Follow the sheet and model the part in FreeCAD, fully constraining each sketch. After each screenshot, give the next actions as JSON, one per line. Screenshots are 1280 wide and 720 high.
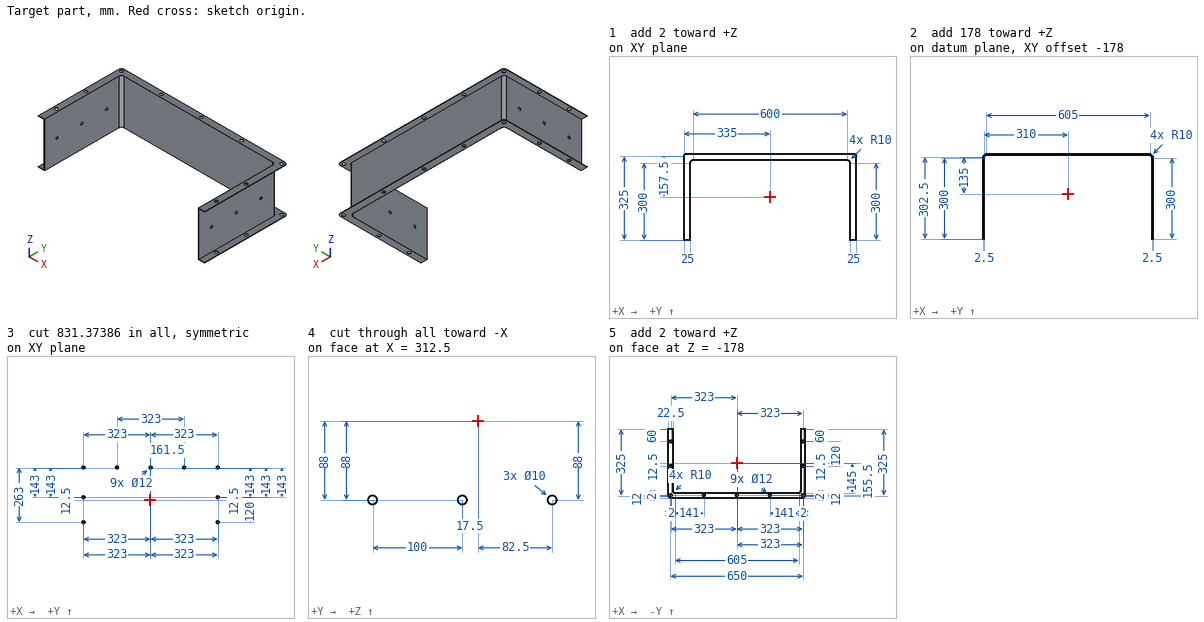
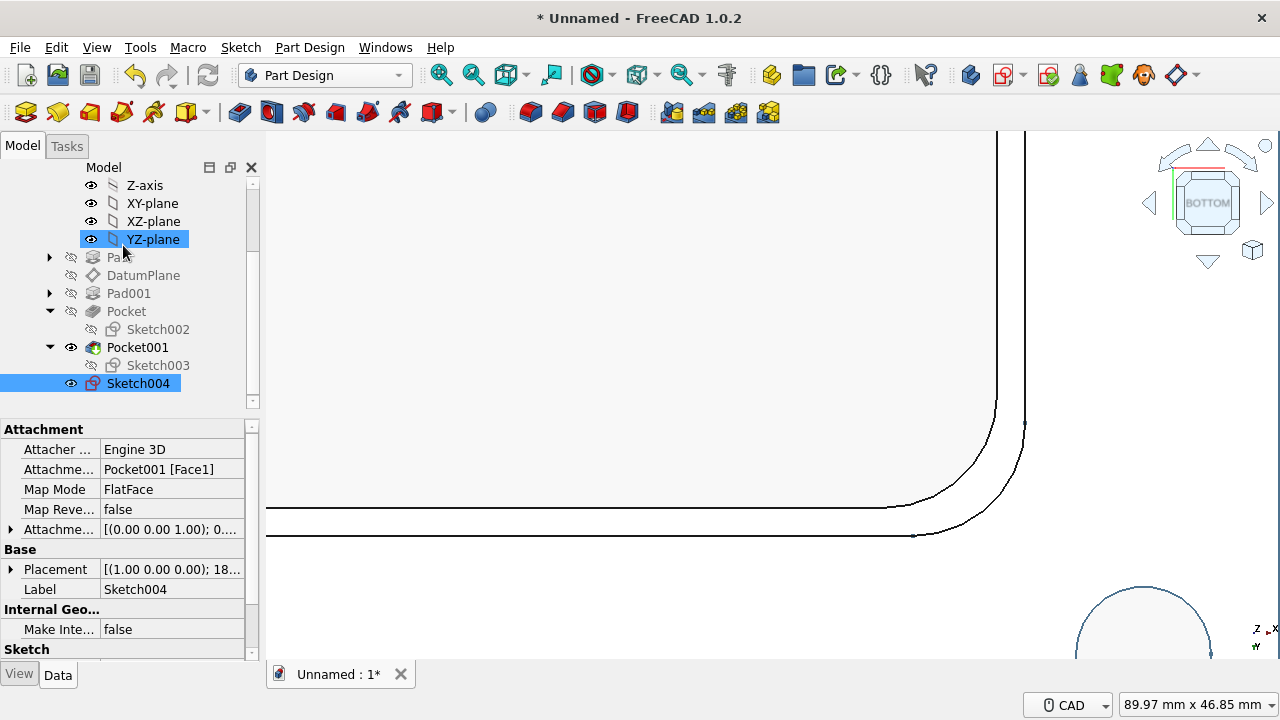
{"action": "left_click", "coordinate": [26, 112]}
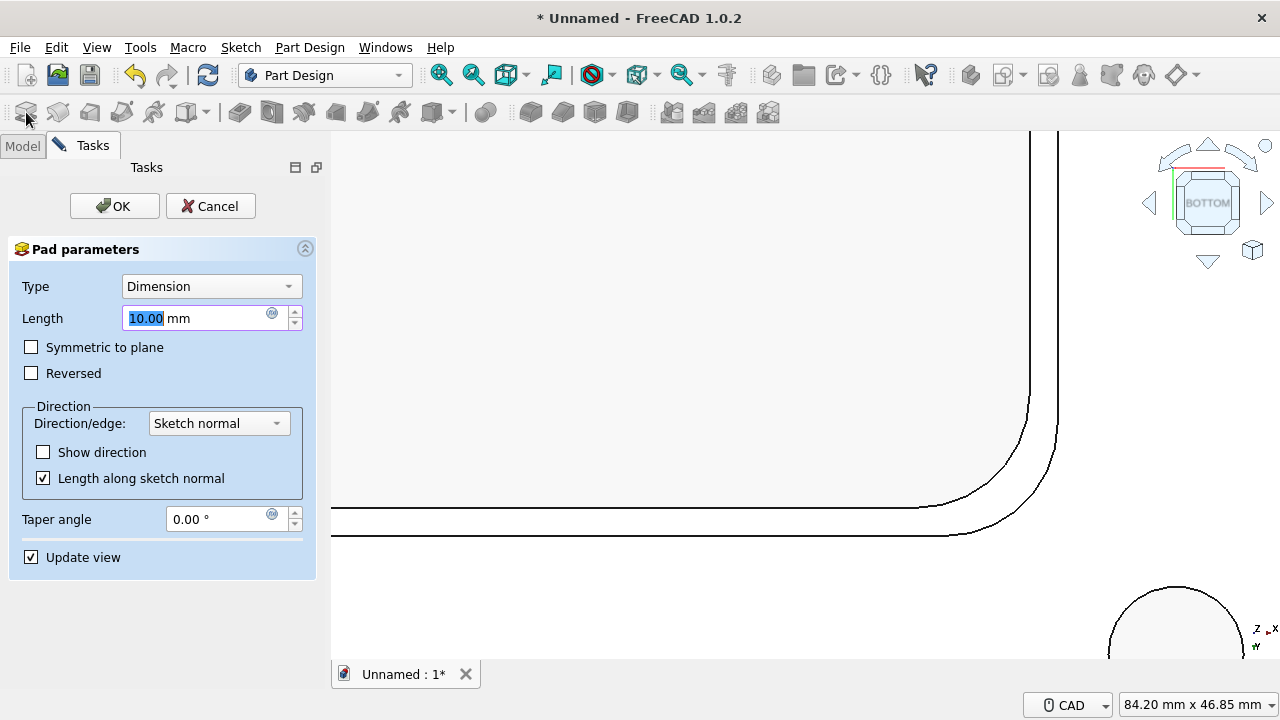
{"action": "type", "text": "2"}
{"action": "key", "text": "Tab"}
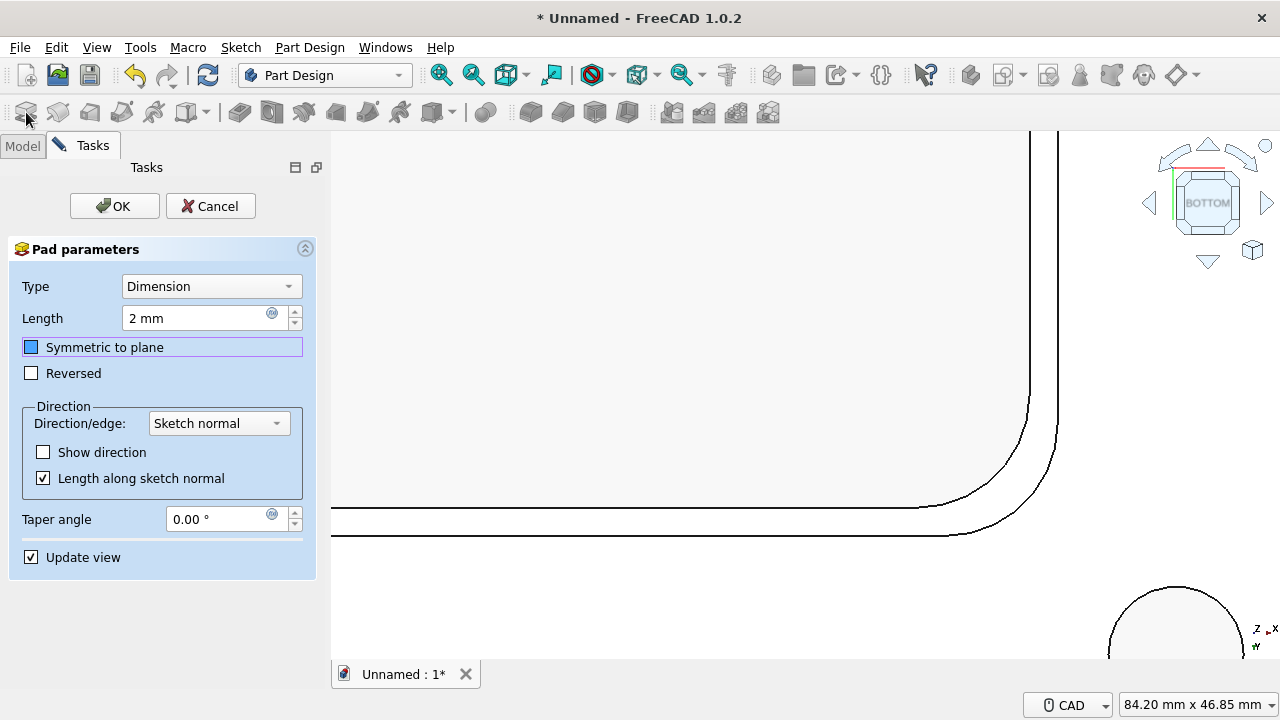
{"action": "left_click", "coordinate": [30, 373]}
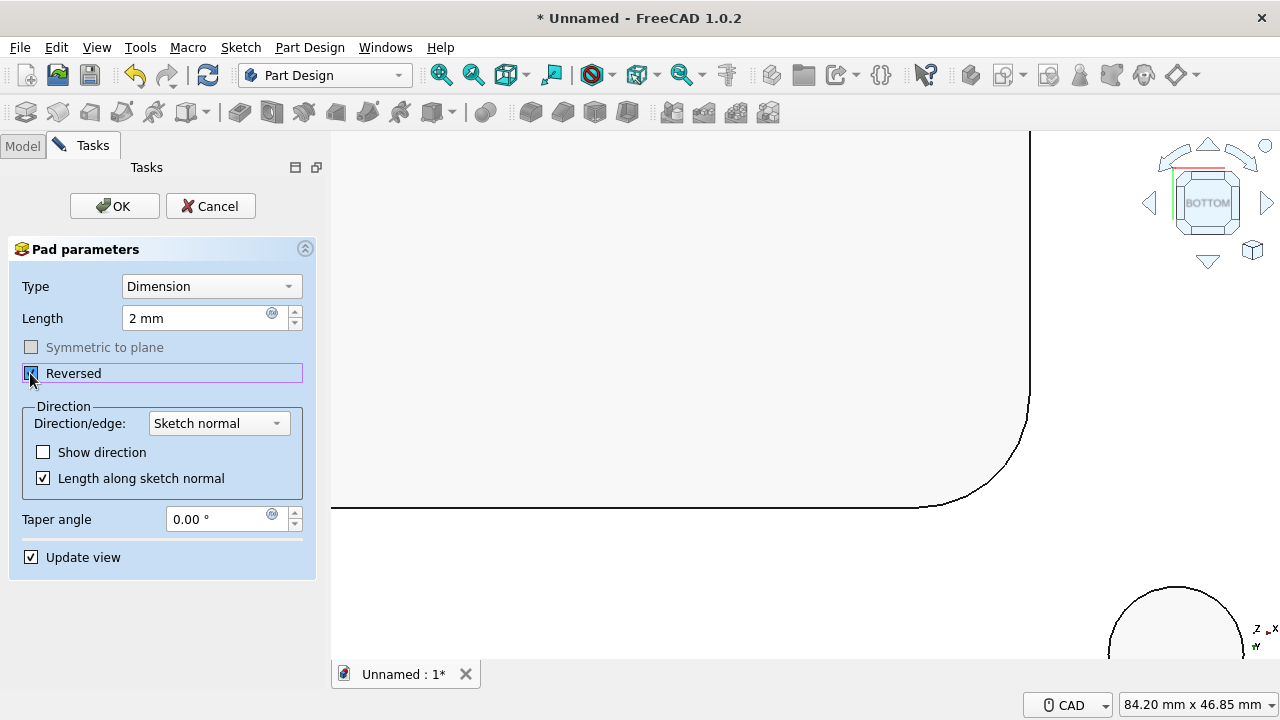
{"action": "left_click", "coordinate": [115, 206]}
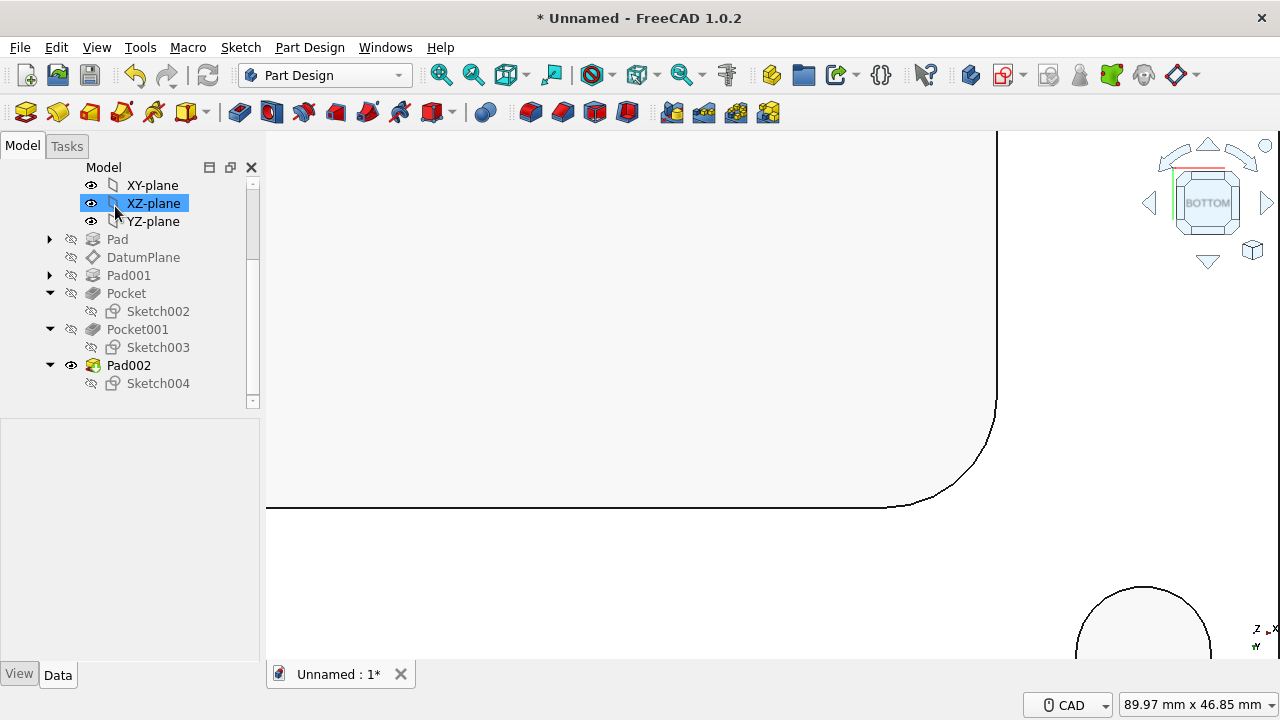
{"action": "key", "text": "0"}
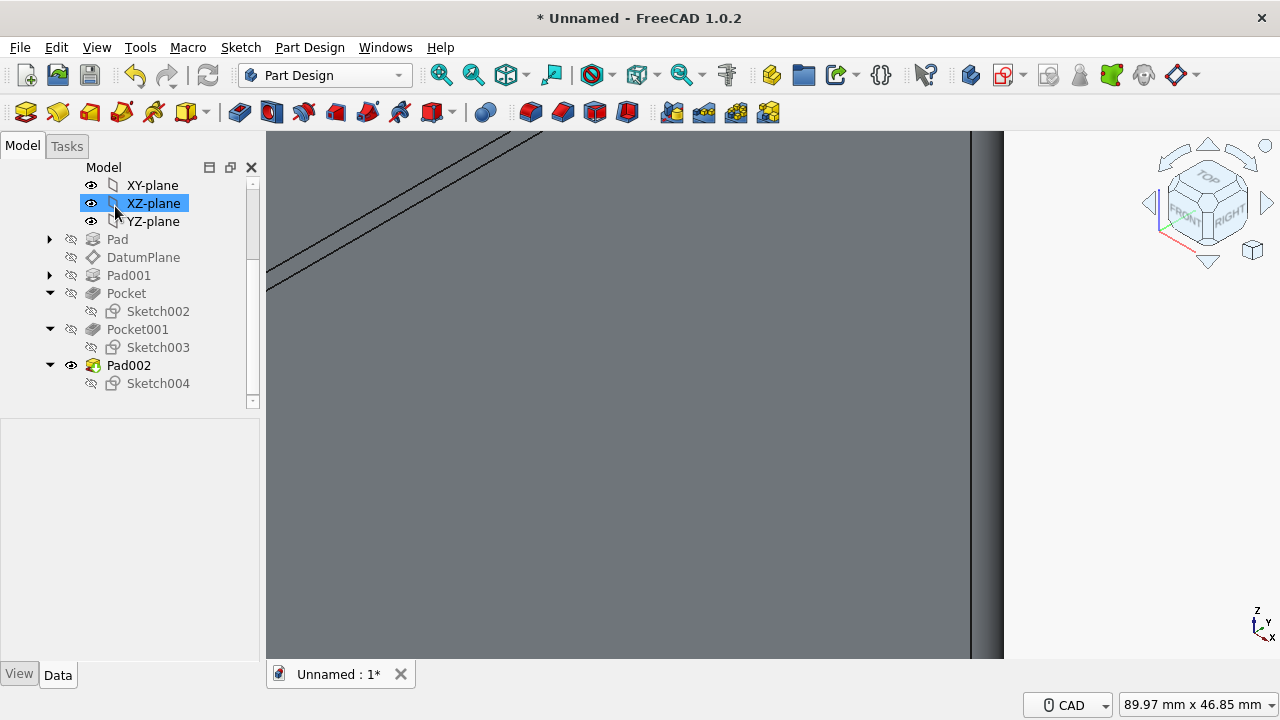
{"action": "left_click", "coordinate": [442, 76]}